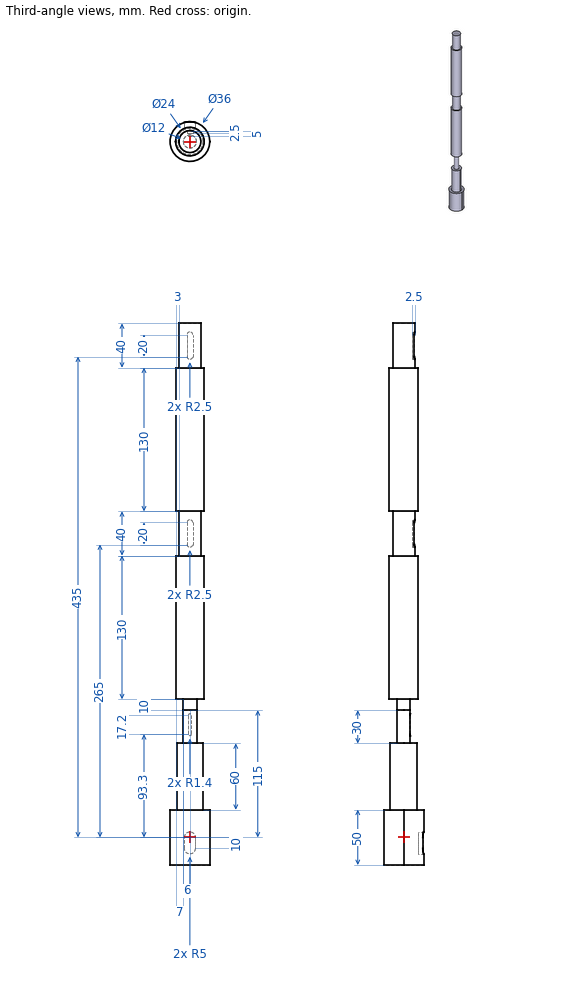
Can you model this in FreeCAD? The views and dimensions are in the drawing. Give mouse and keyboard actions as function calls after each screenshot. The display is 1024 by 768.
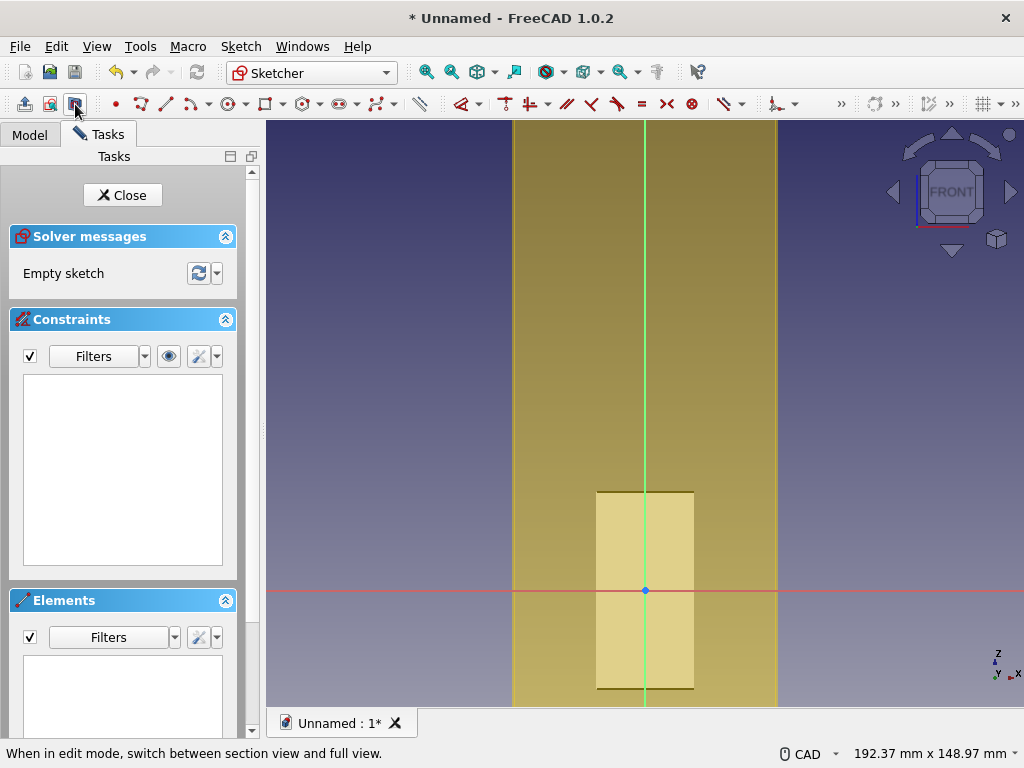
scroll(662, 660, up, 8)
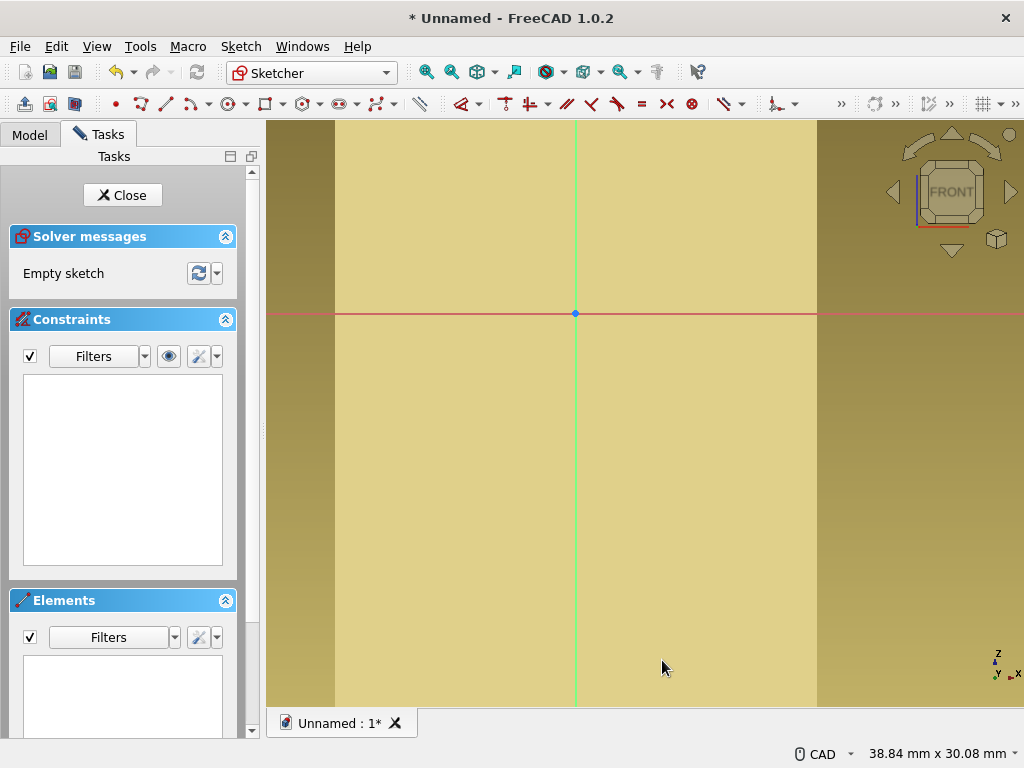
click(338, 104)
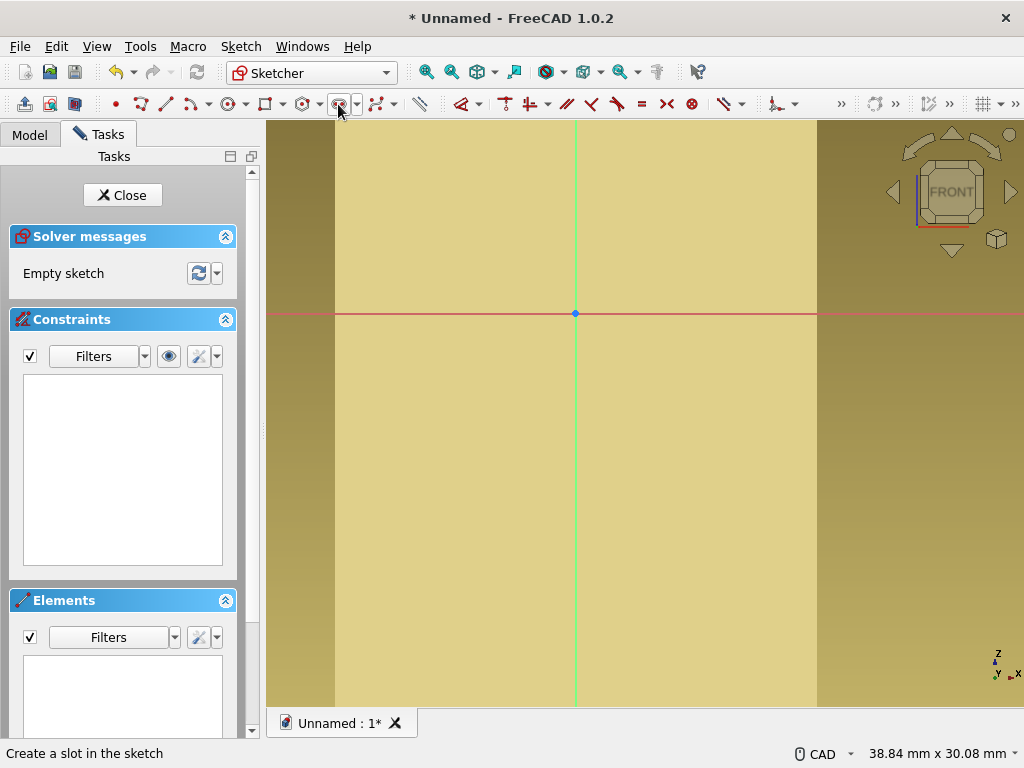
click(576, 314)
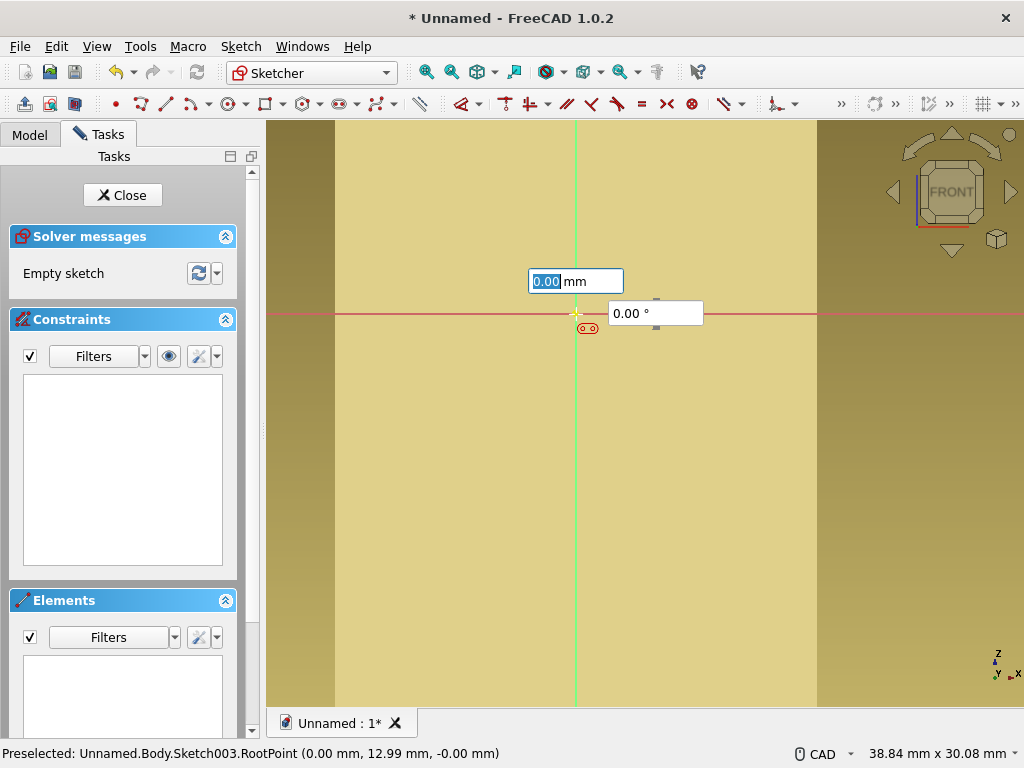
click(585, 509)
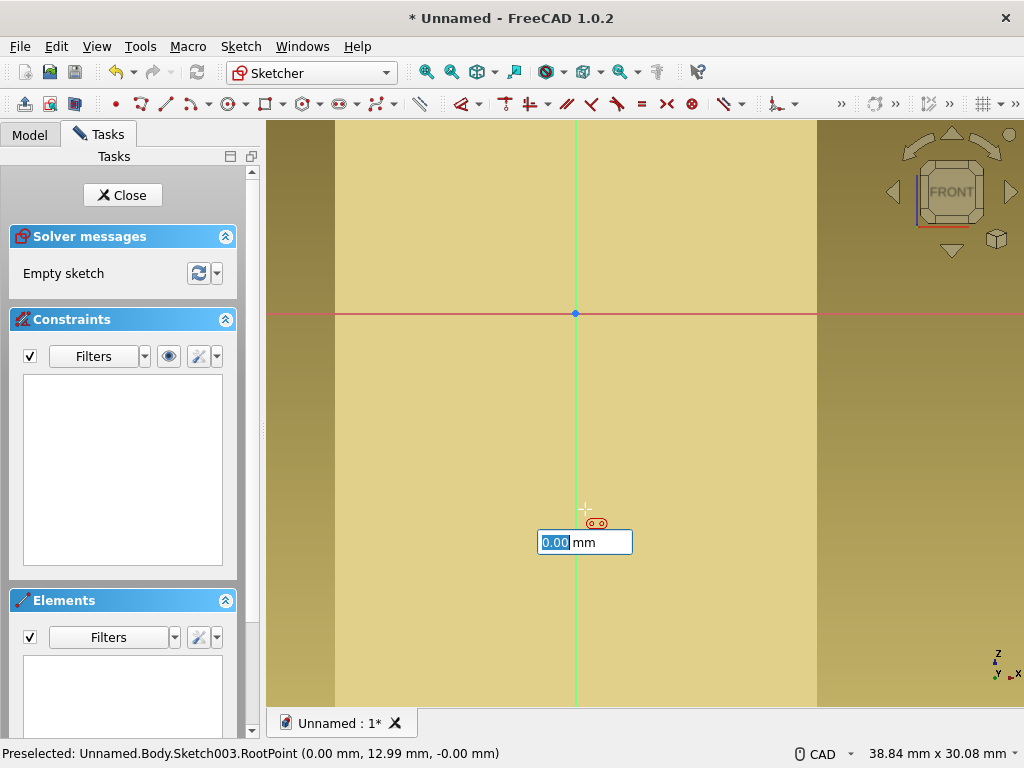
click(673, 411)
key(Escape)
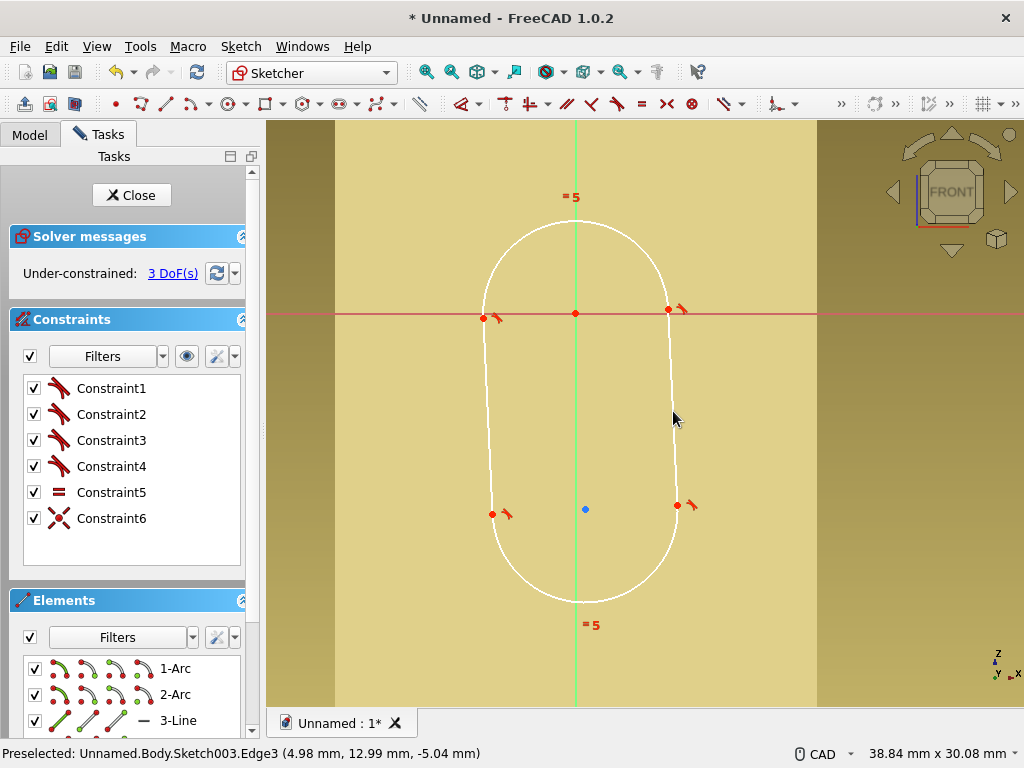
click(671, 368)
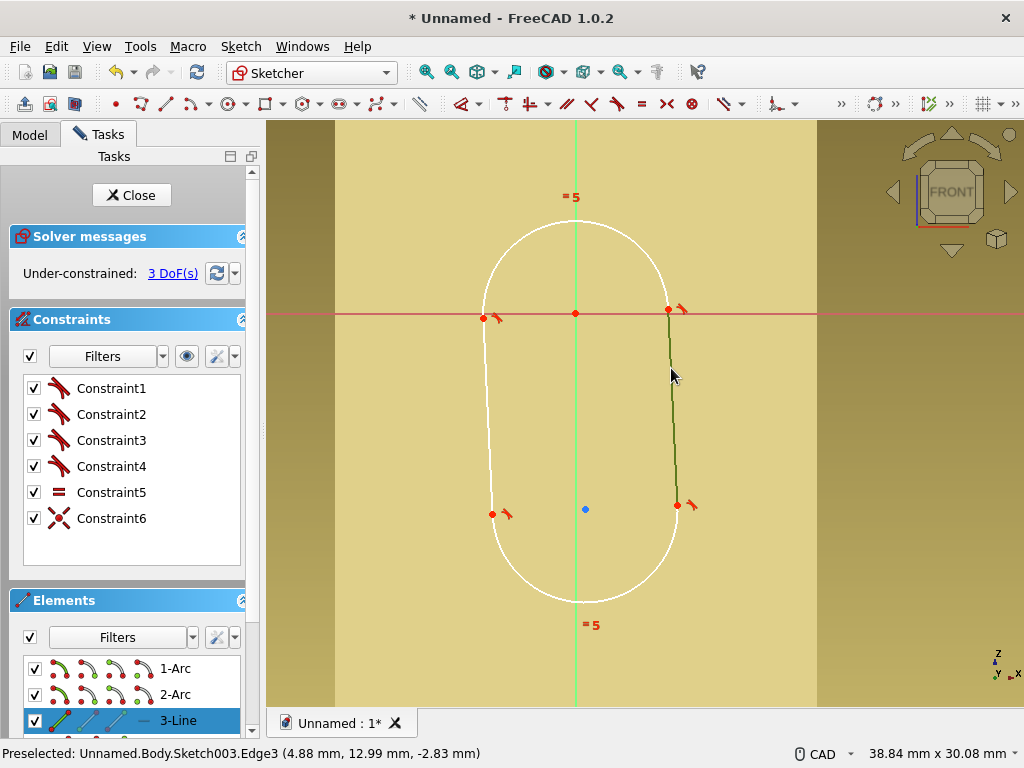
key(v)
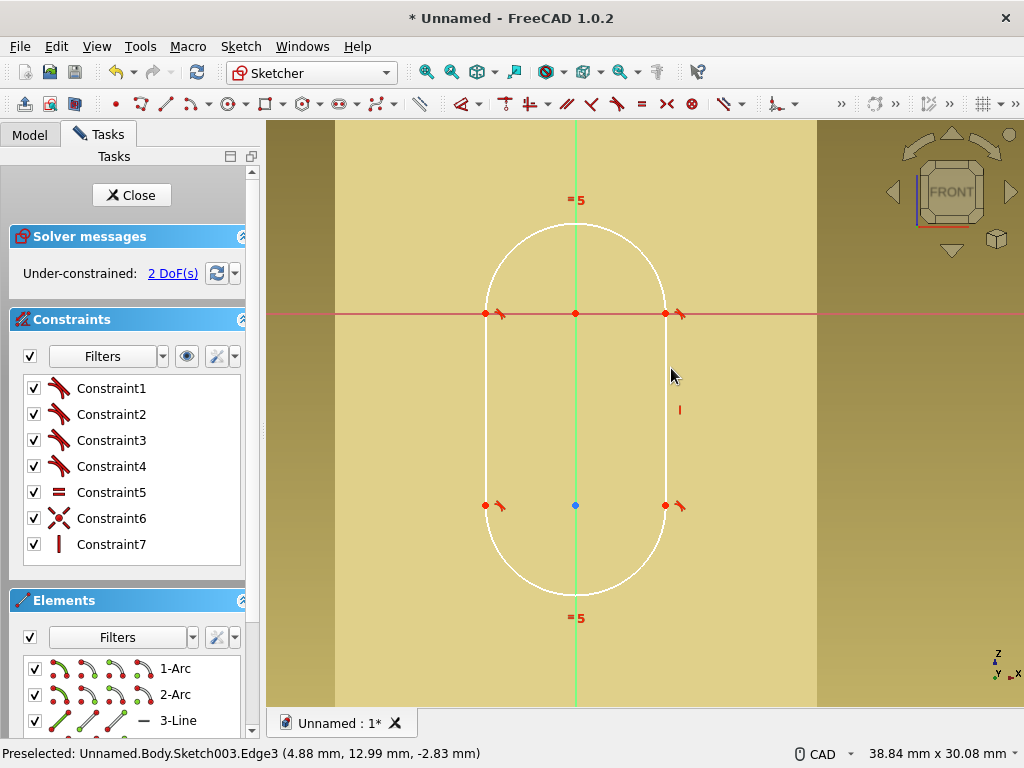
click(460, 104)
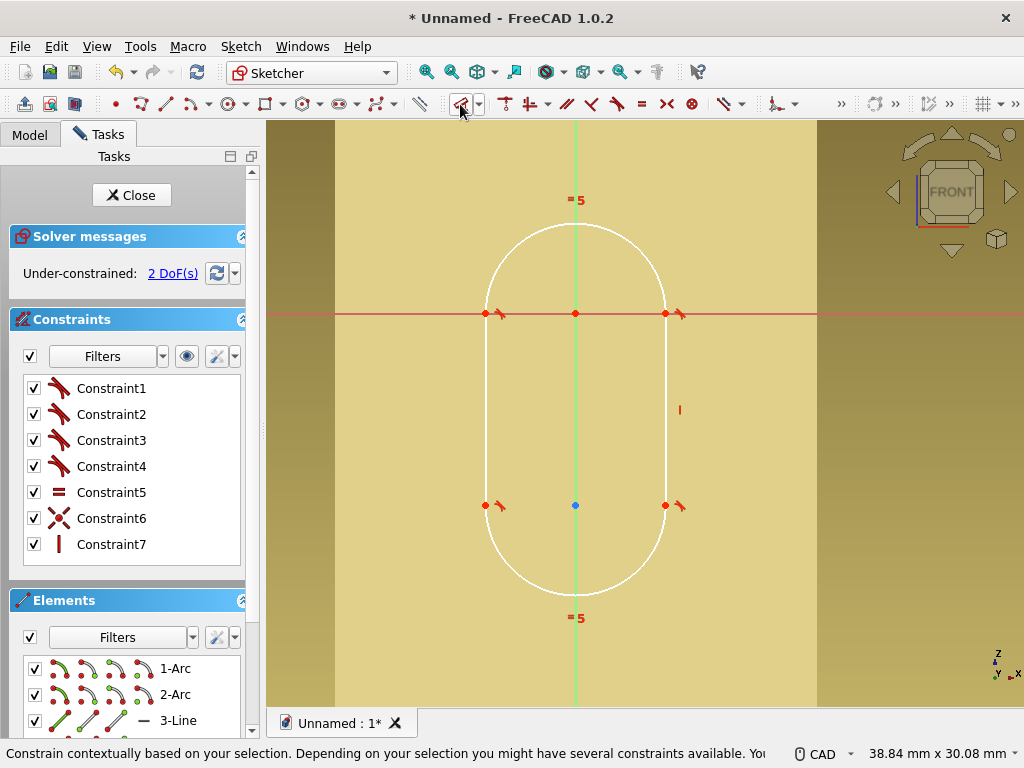
click(629, 241)
click(648, 215)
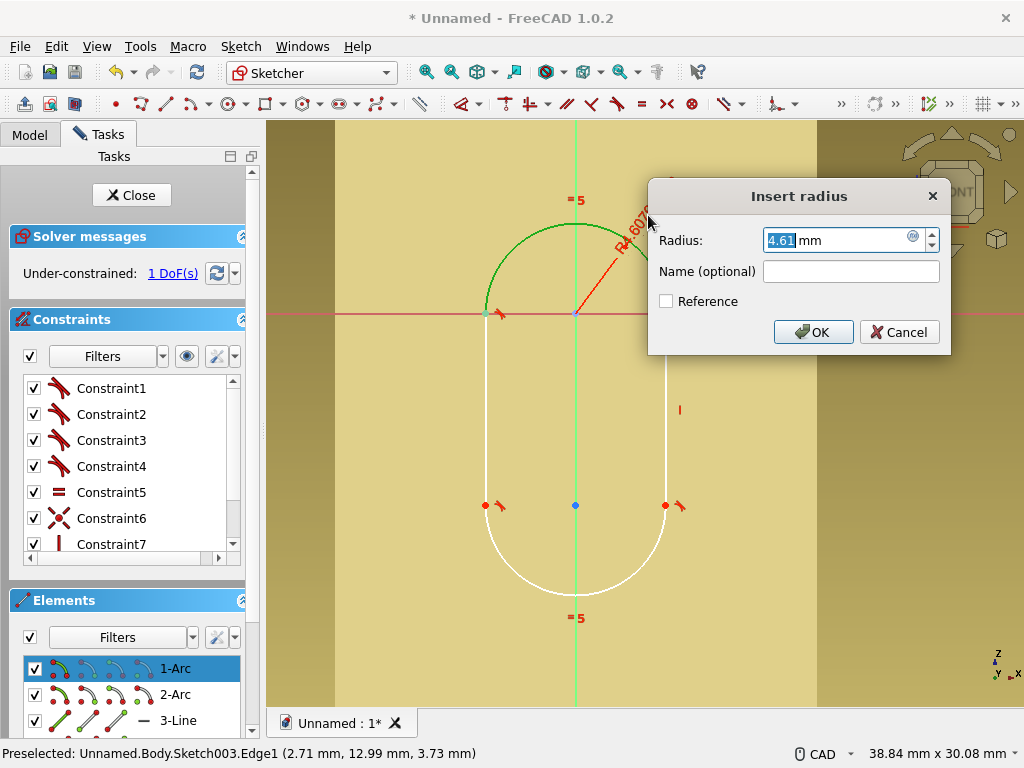
text(5)
key(Return)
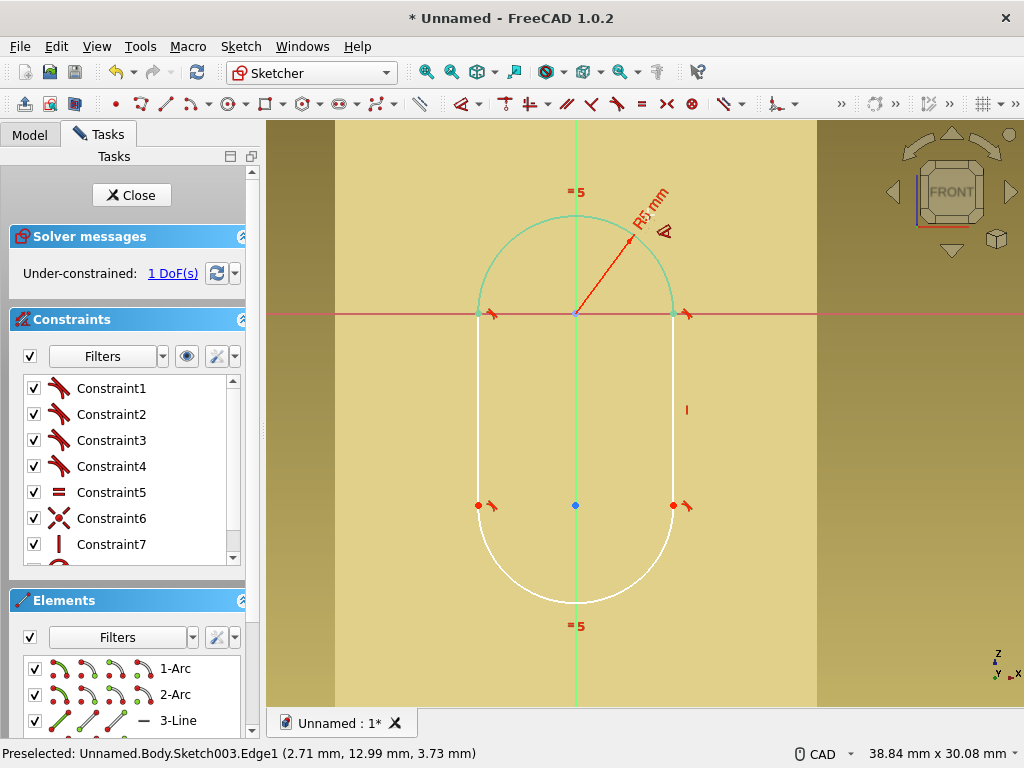
click(673, 371)
click(707, 410)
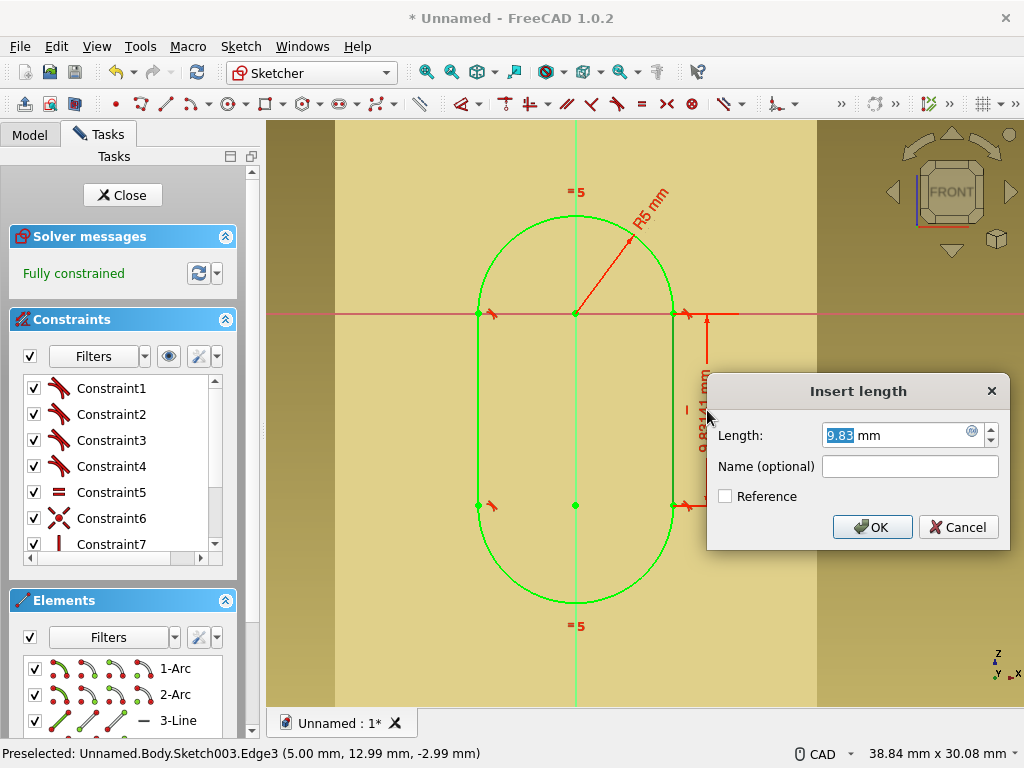
text(10)
key(Return)
key(Escape)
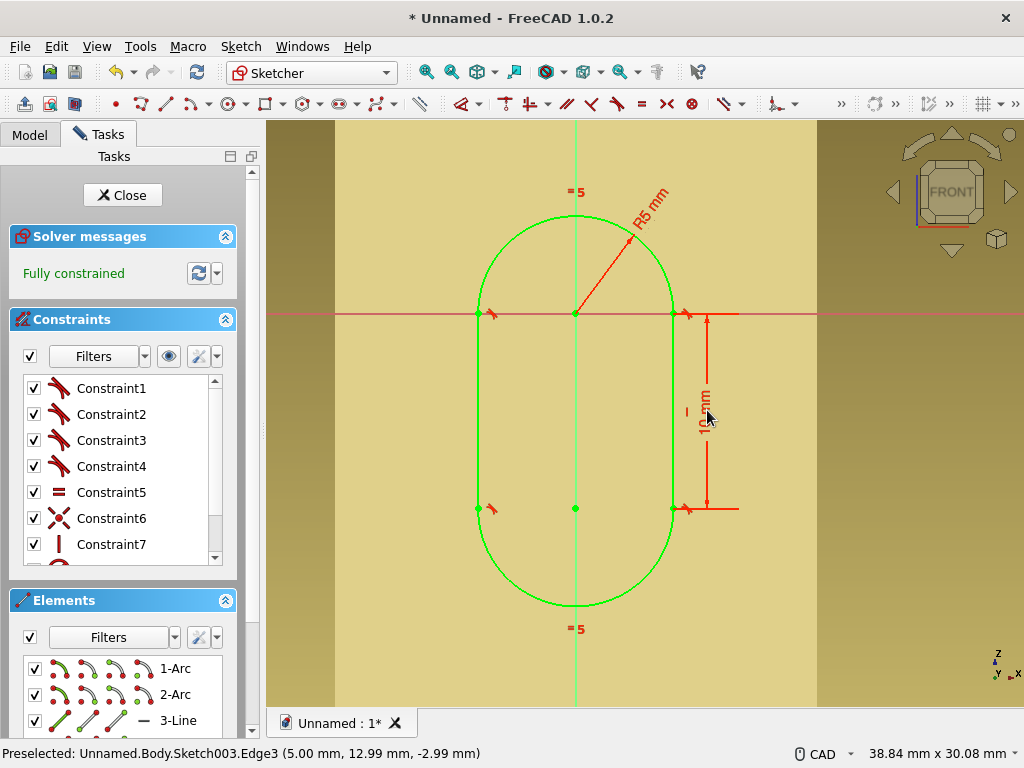
click(123, 195)